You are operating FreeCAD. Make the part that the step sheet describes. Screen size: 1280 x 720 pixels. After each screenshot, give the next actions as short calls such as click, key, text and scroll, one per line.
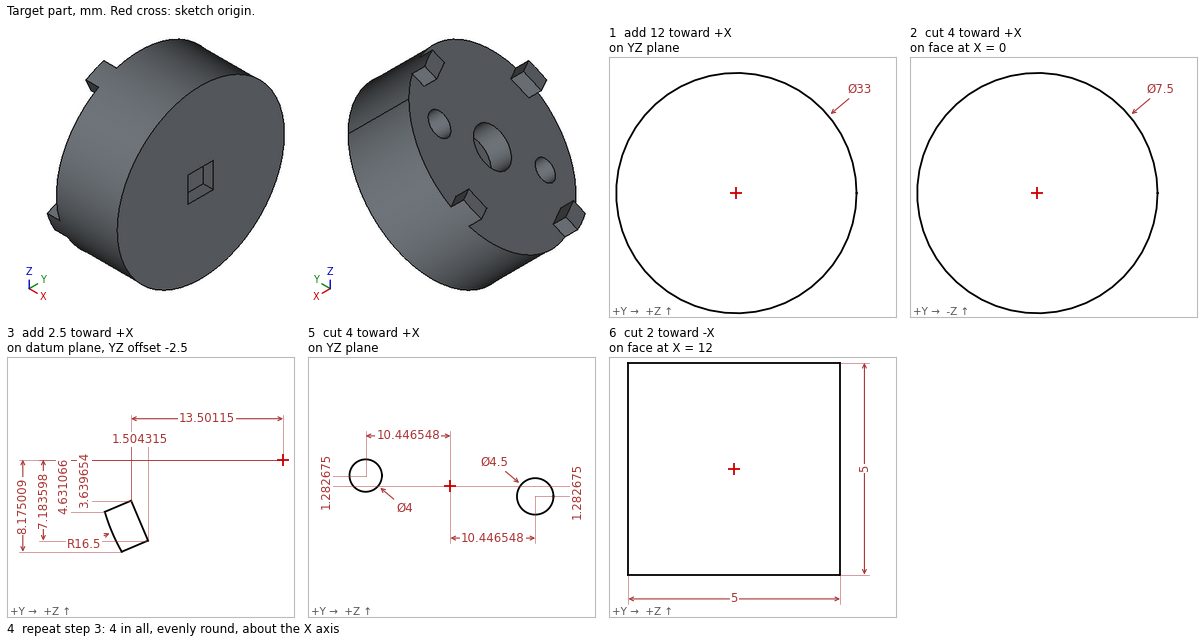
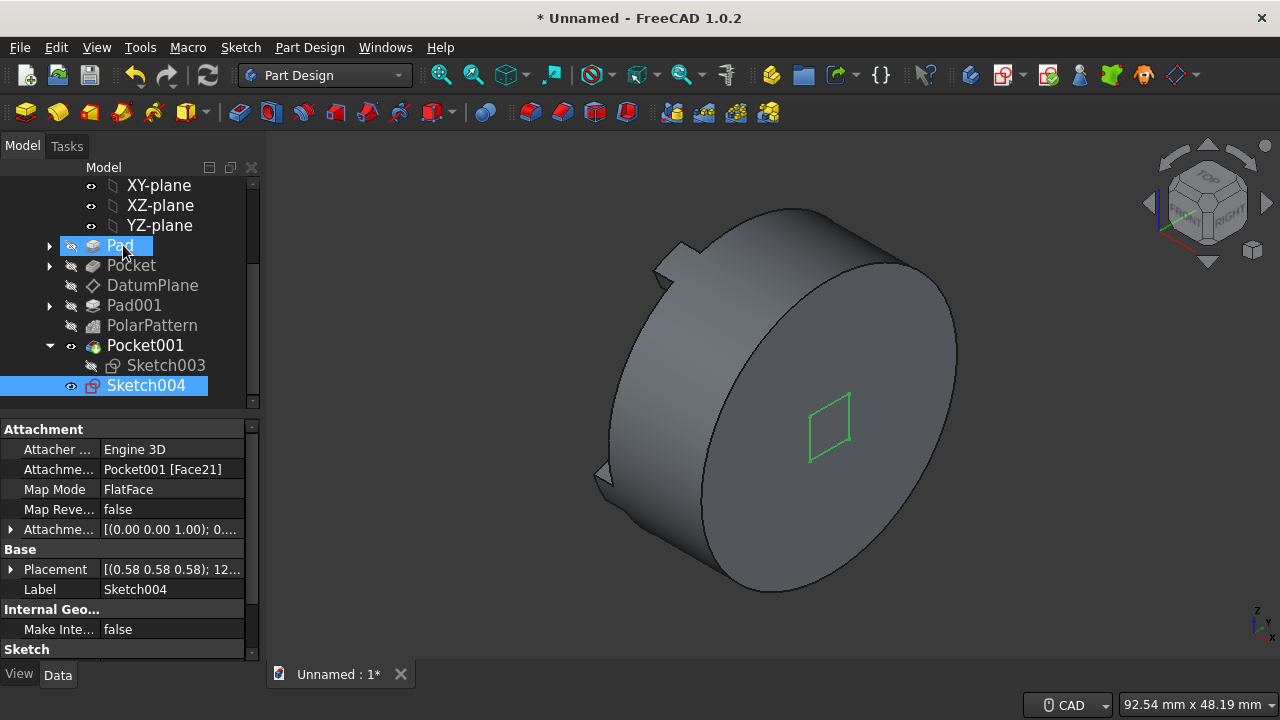
click(240, 112)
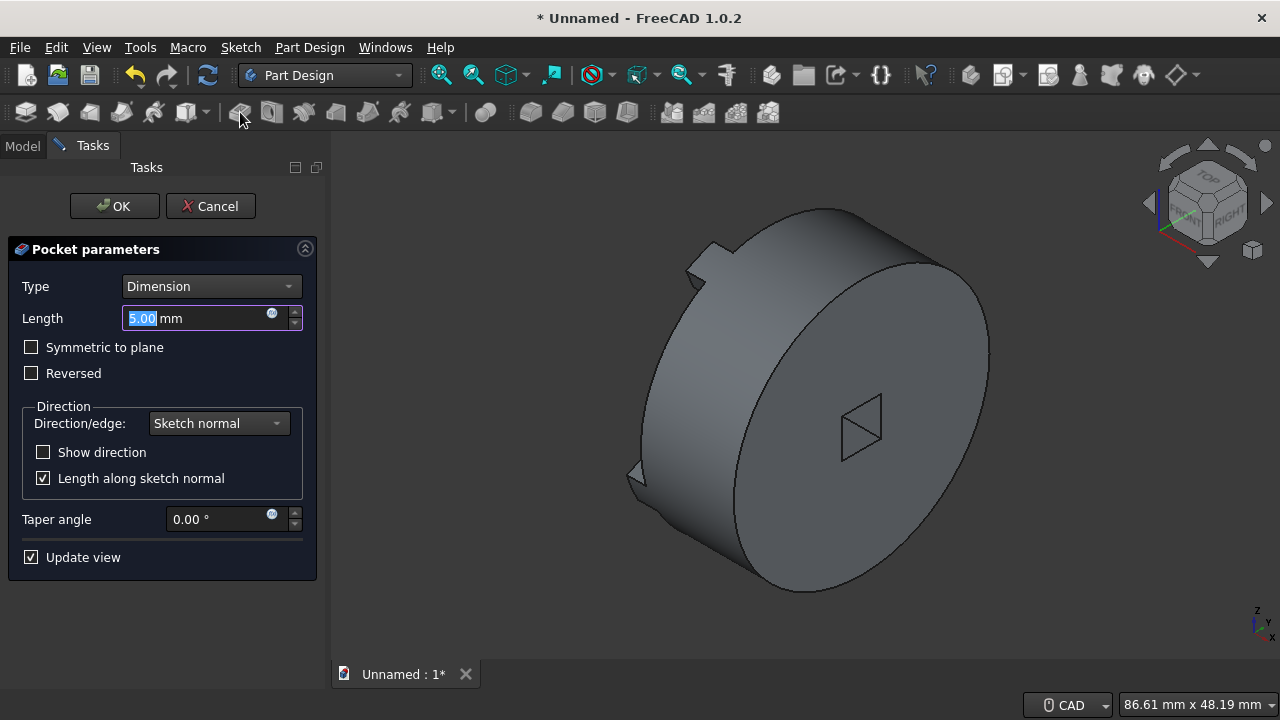
text(2)
key(Tab)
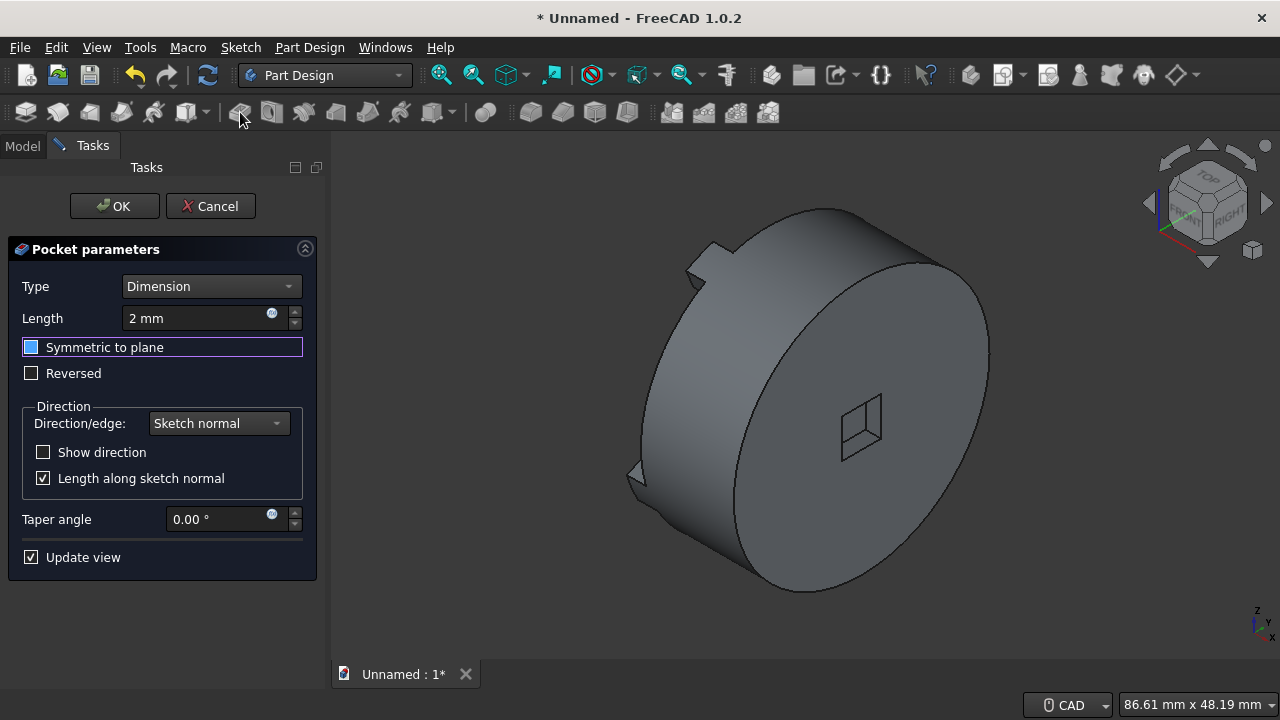
click(115, 206)